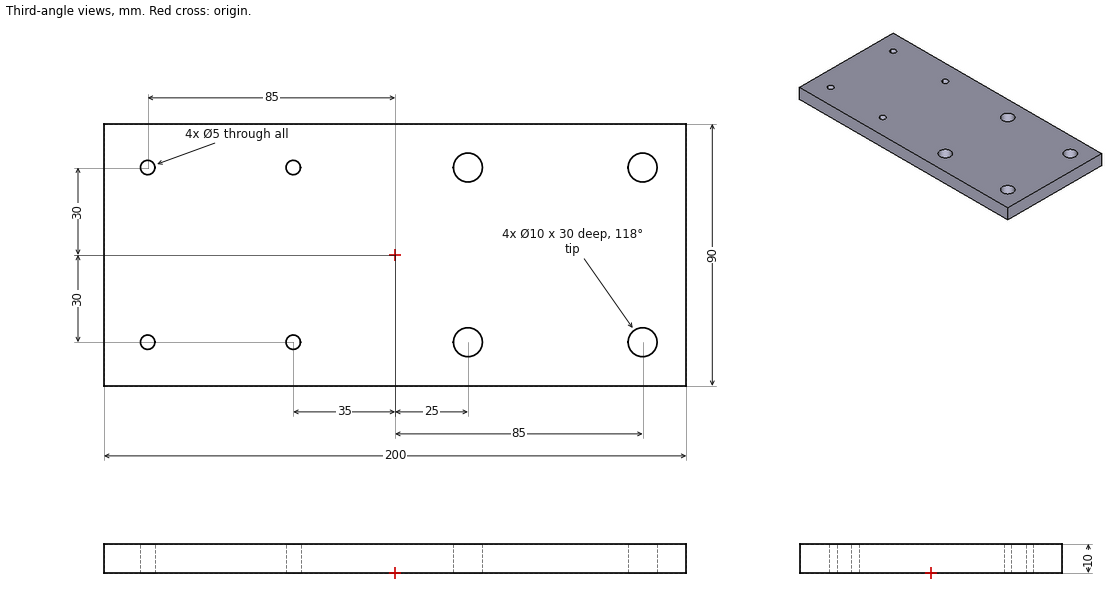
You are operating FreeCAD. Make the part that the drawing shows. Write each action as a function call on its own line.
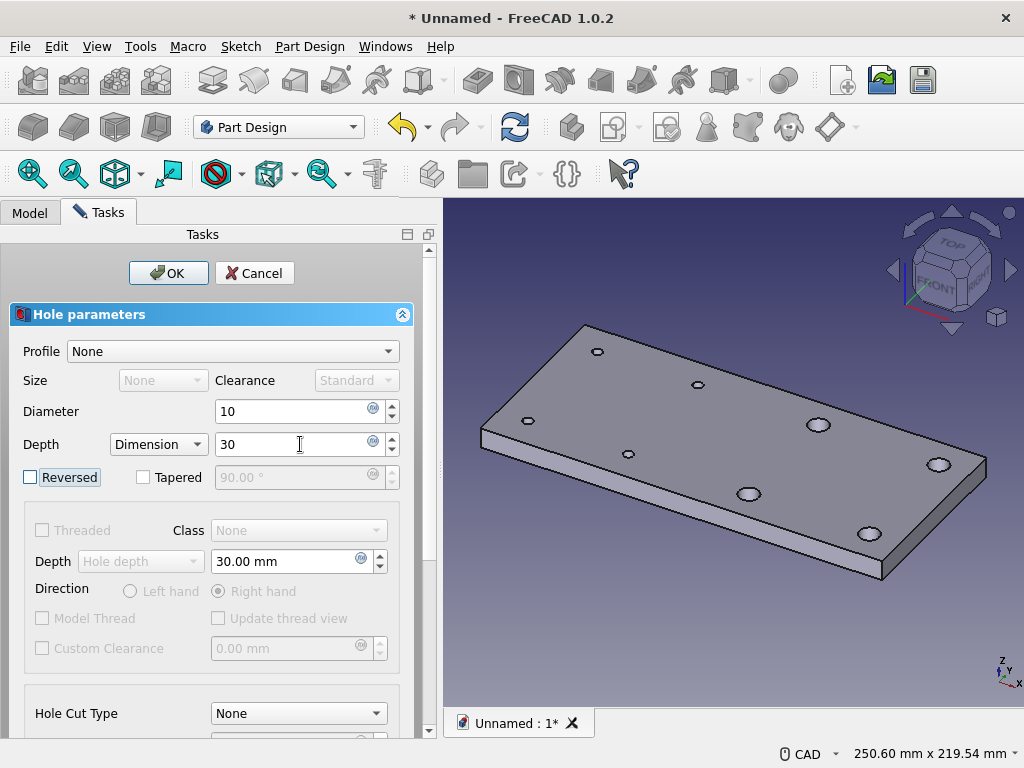
click(169, 273)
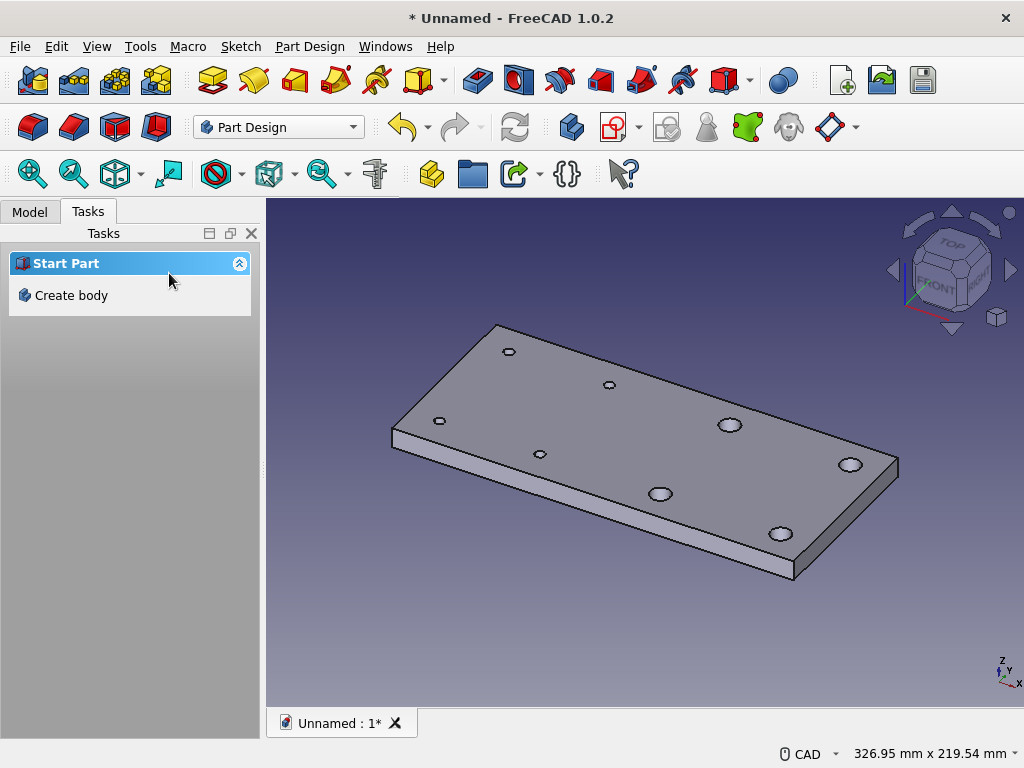
key(0)